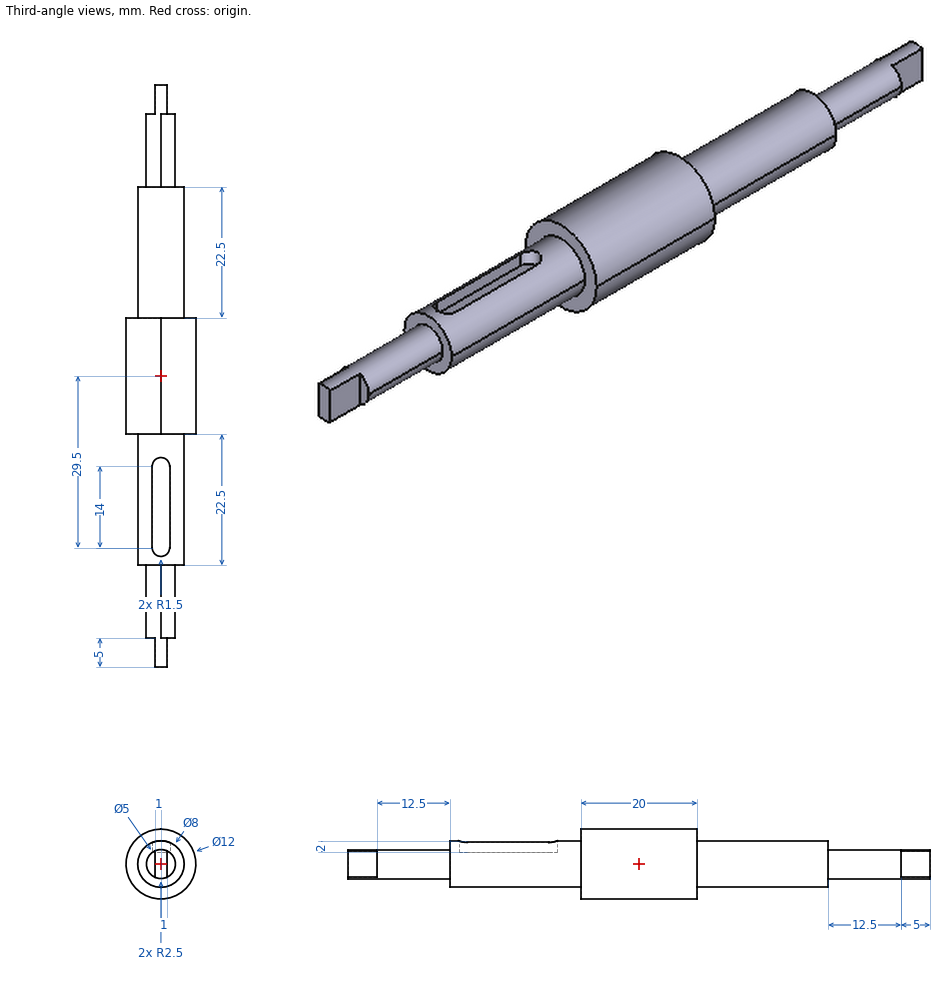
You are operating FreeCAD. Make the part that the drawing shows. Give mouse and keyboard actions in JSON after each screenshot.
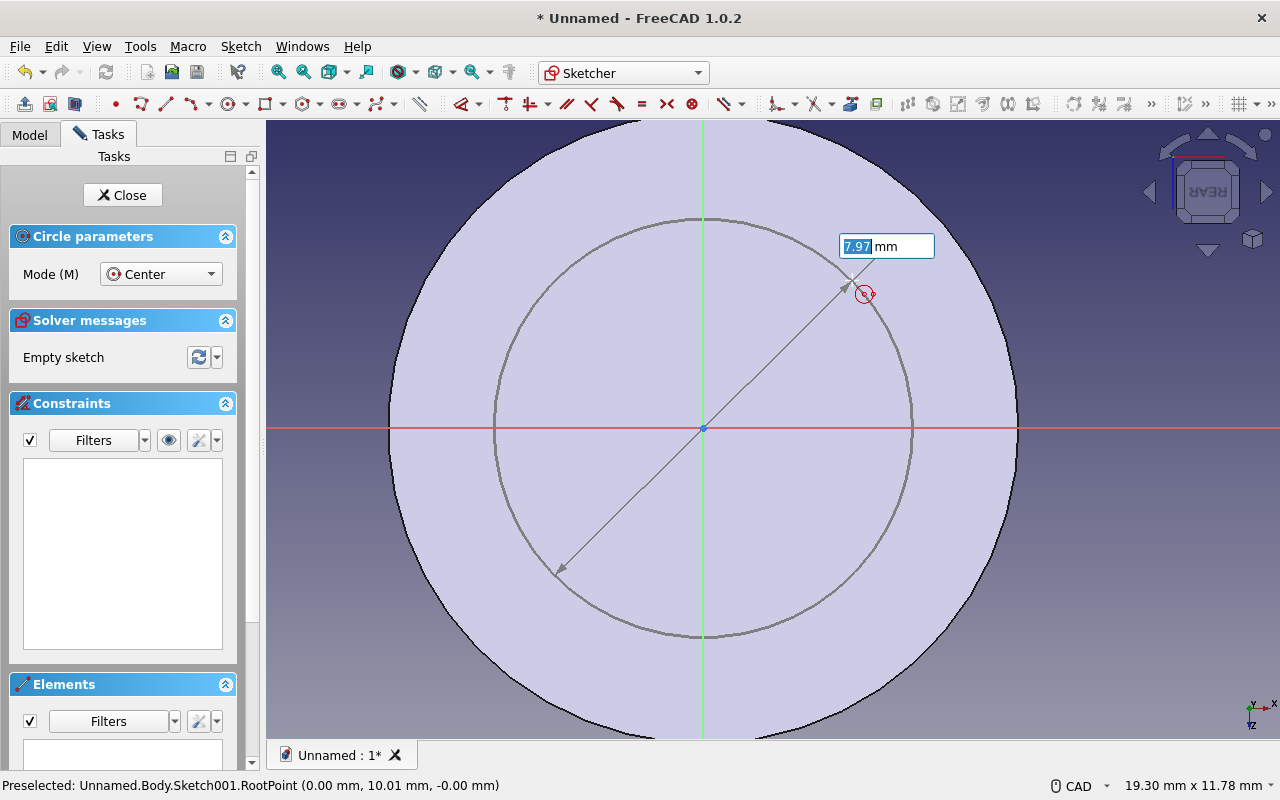
{"action": "type", "text": "8"}
{"action": "key", "text": "Return"}
{"action": "key", "text": "Escape"}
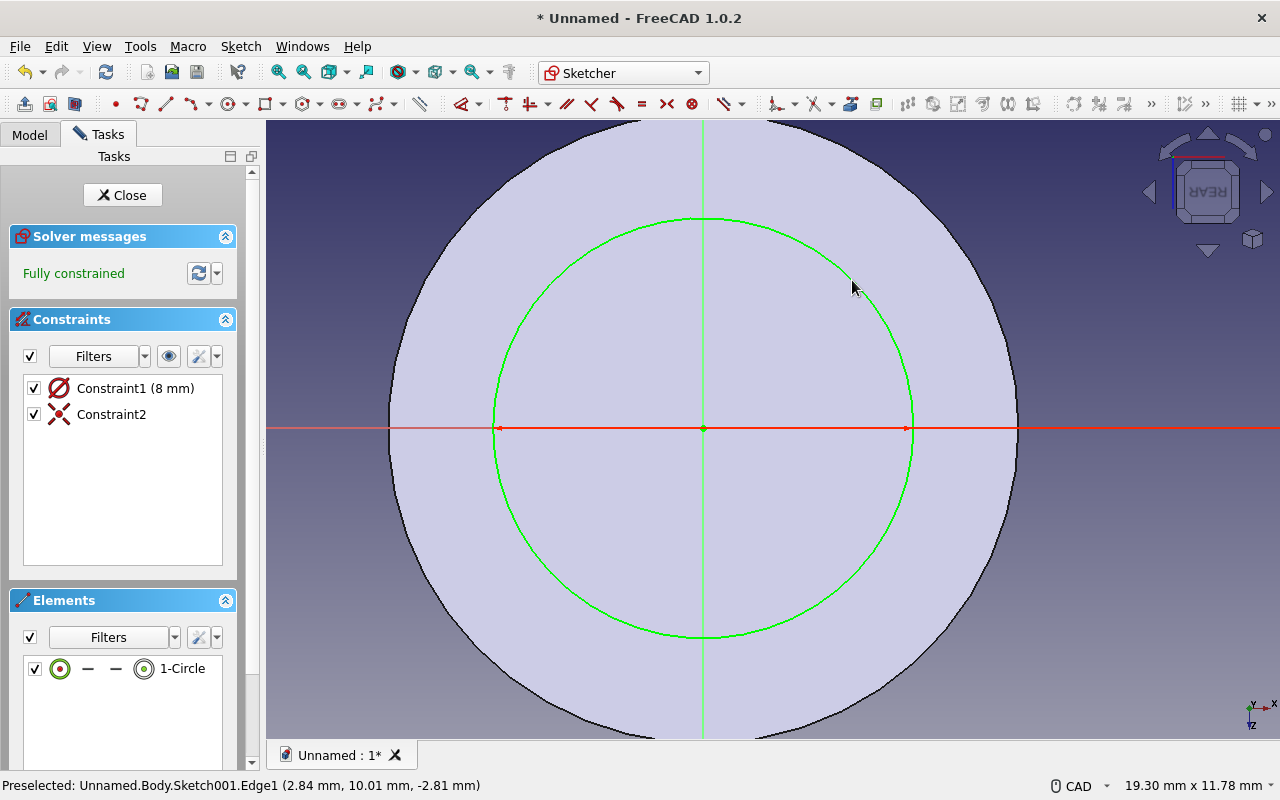
{"action": "left_click", "coordinate": [123, 195]}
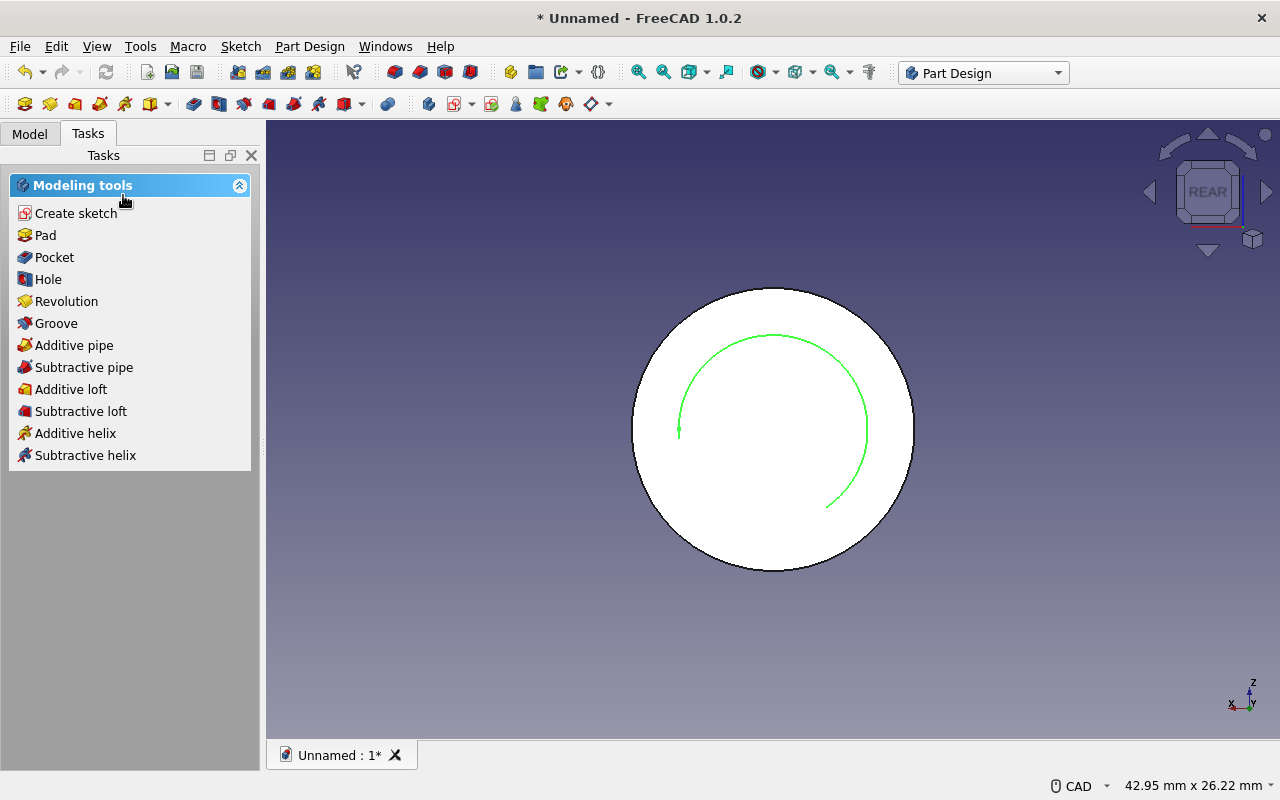
{"action": "left_click", "coordinate": [25, 104]}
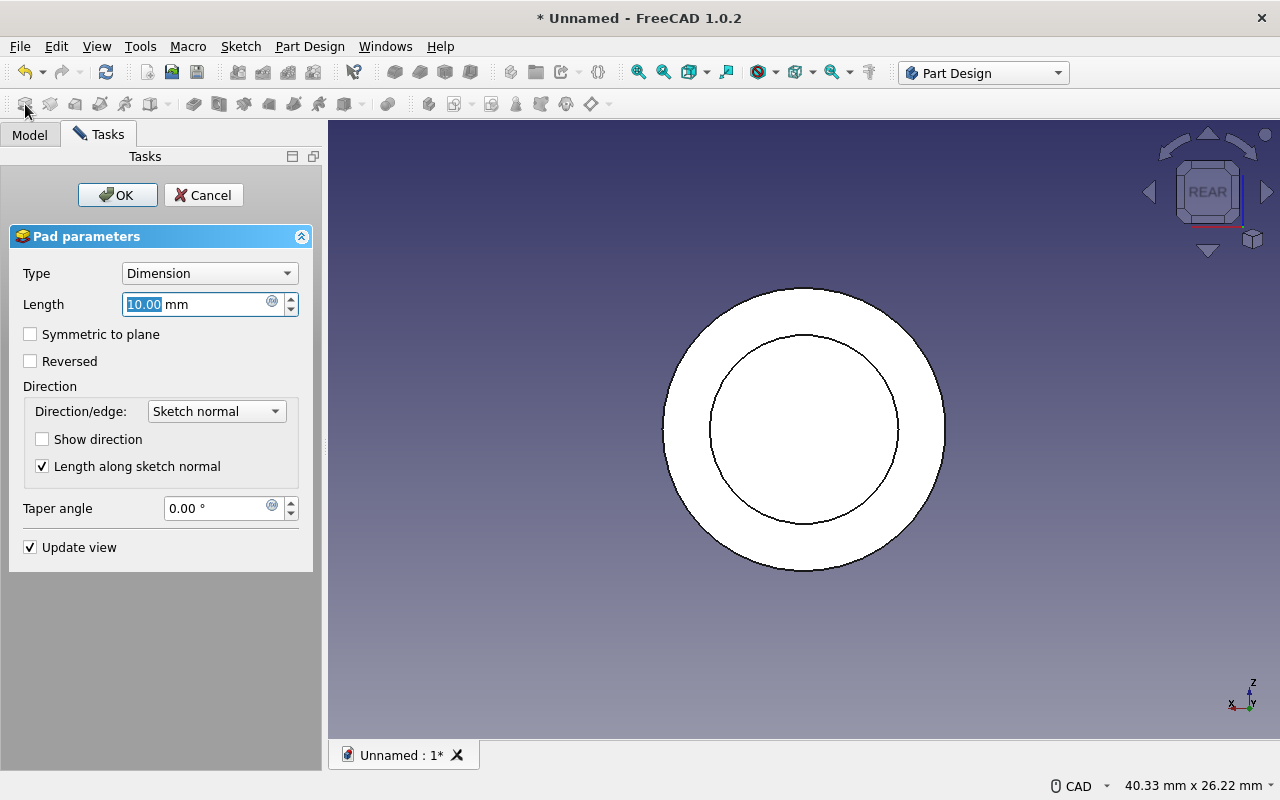
{"action": "type", "text": "22.5"}
{"action": "key", "text": "Tab"}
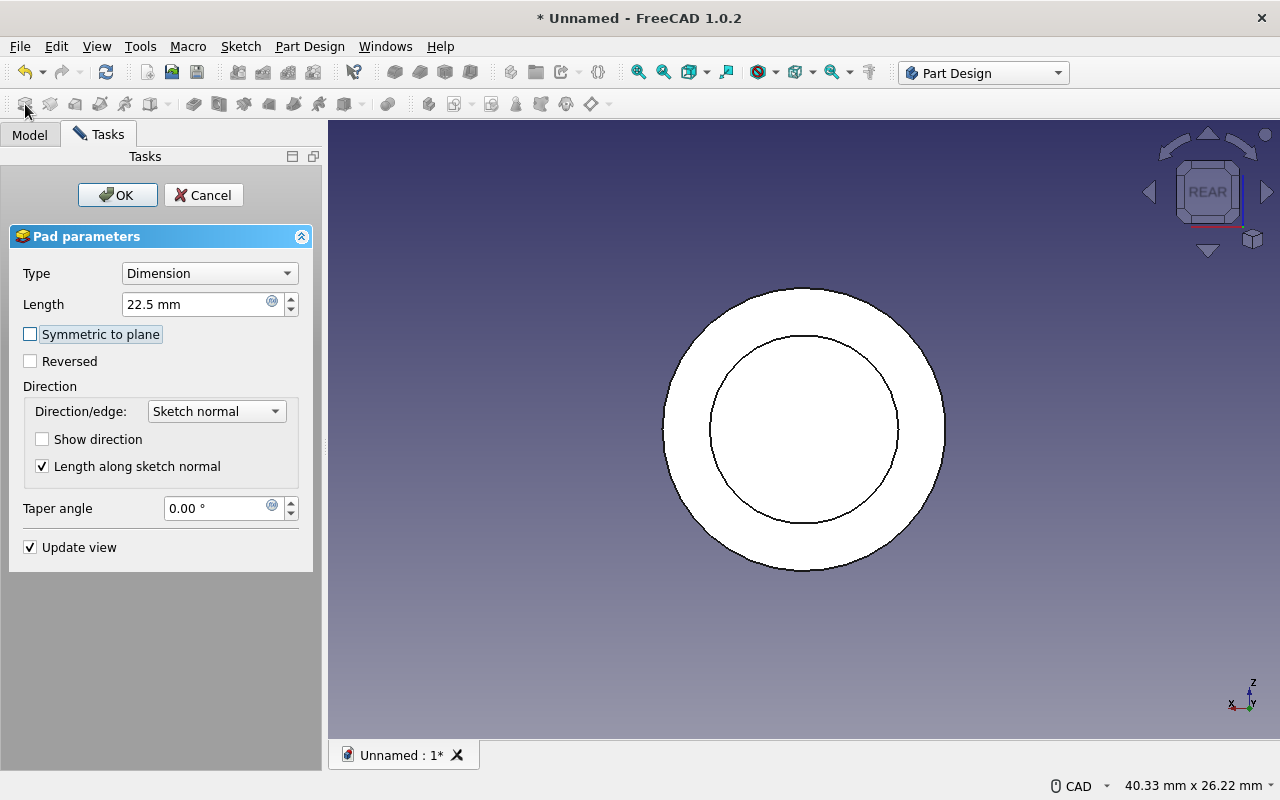
{"action": "left_click", "coordinate": [118, 195]}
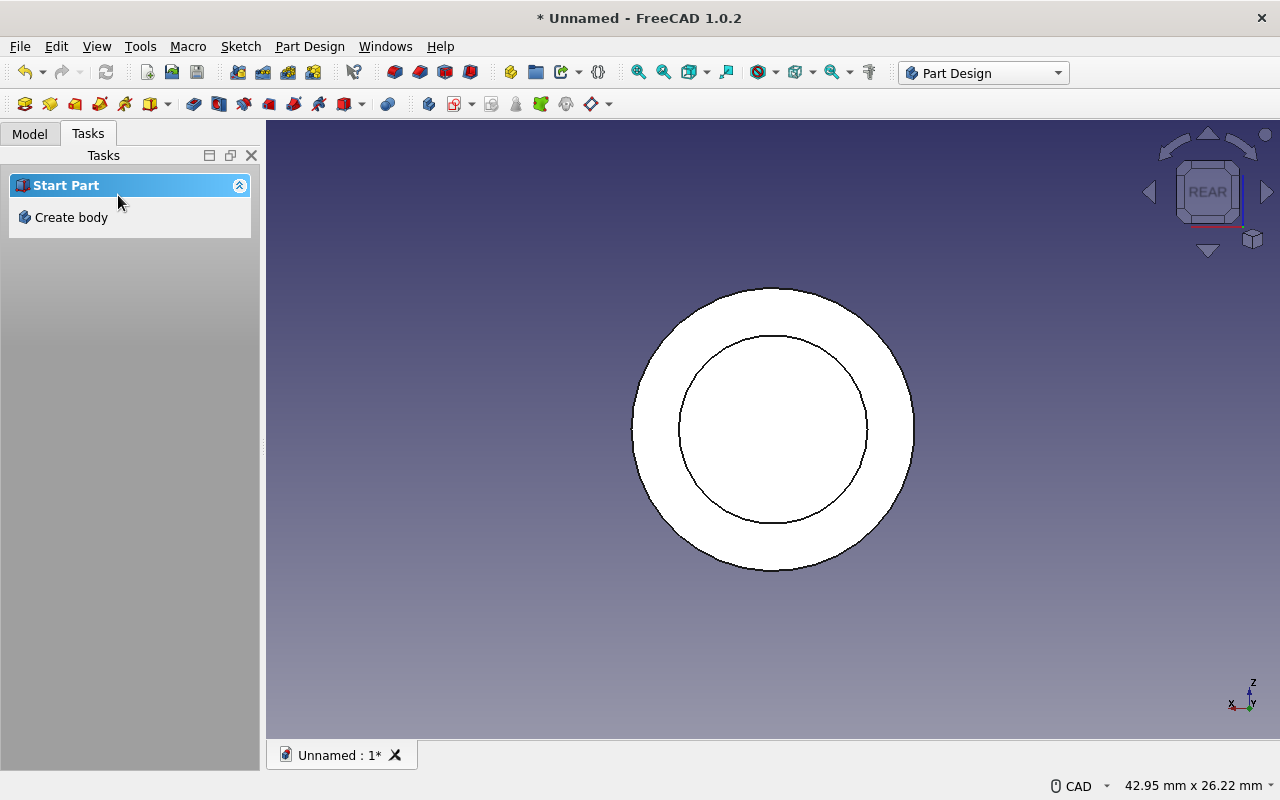
{"action": "left_click", "coordinate": [773, 428]}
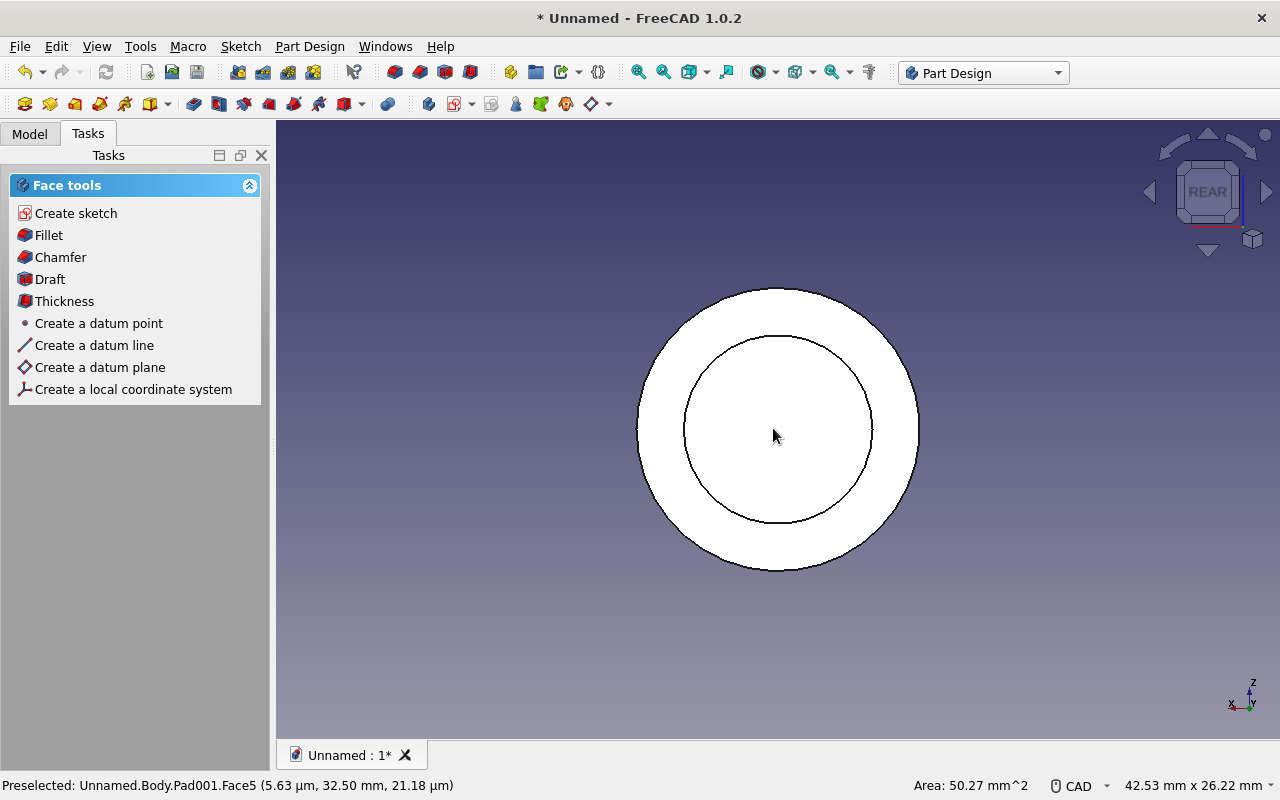
{"action": "left_click", "coordinate": [454, 104]}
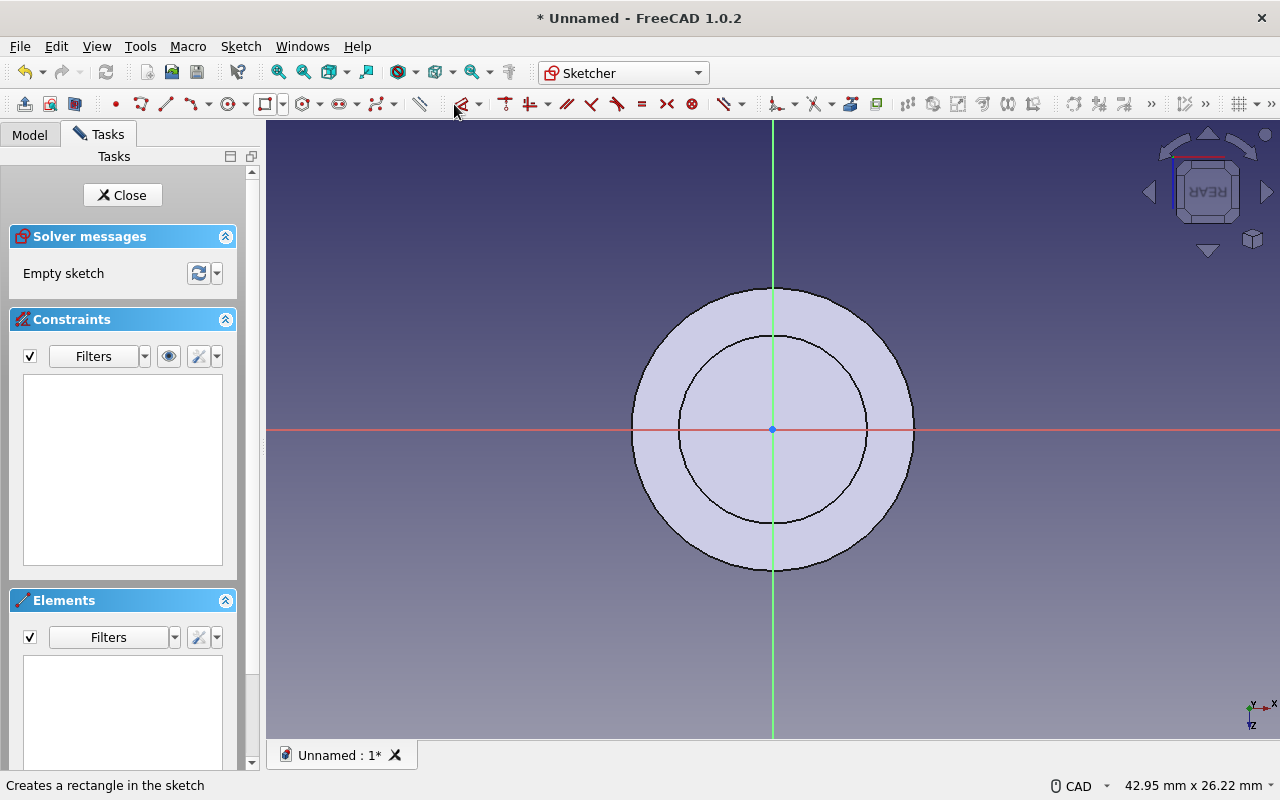
{"action": "scroll", "coordinate": [802, 429], "scroll_direction": "up", "scroll_amount": 6}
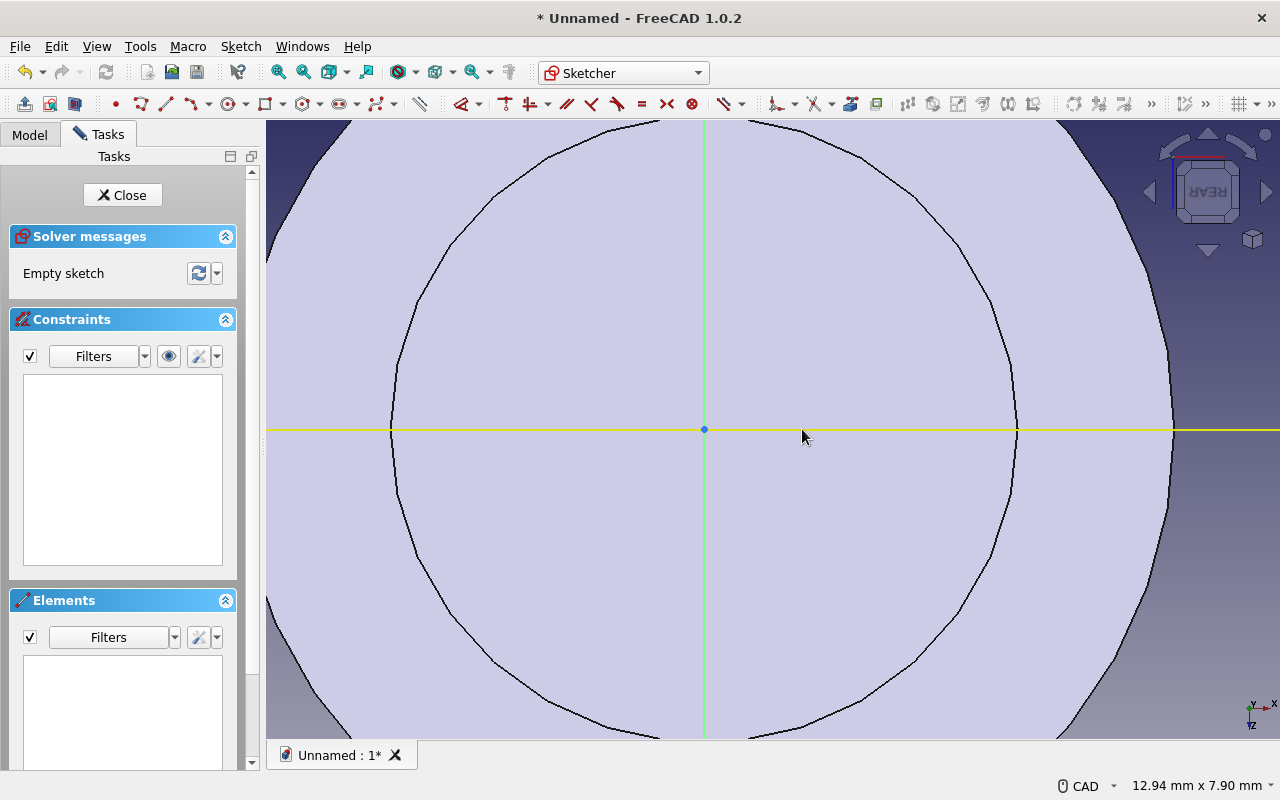
{"action": "key", "text": "g c"}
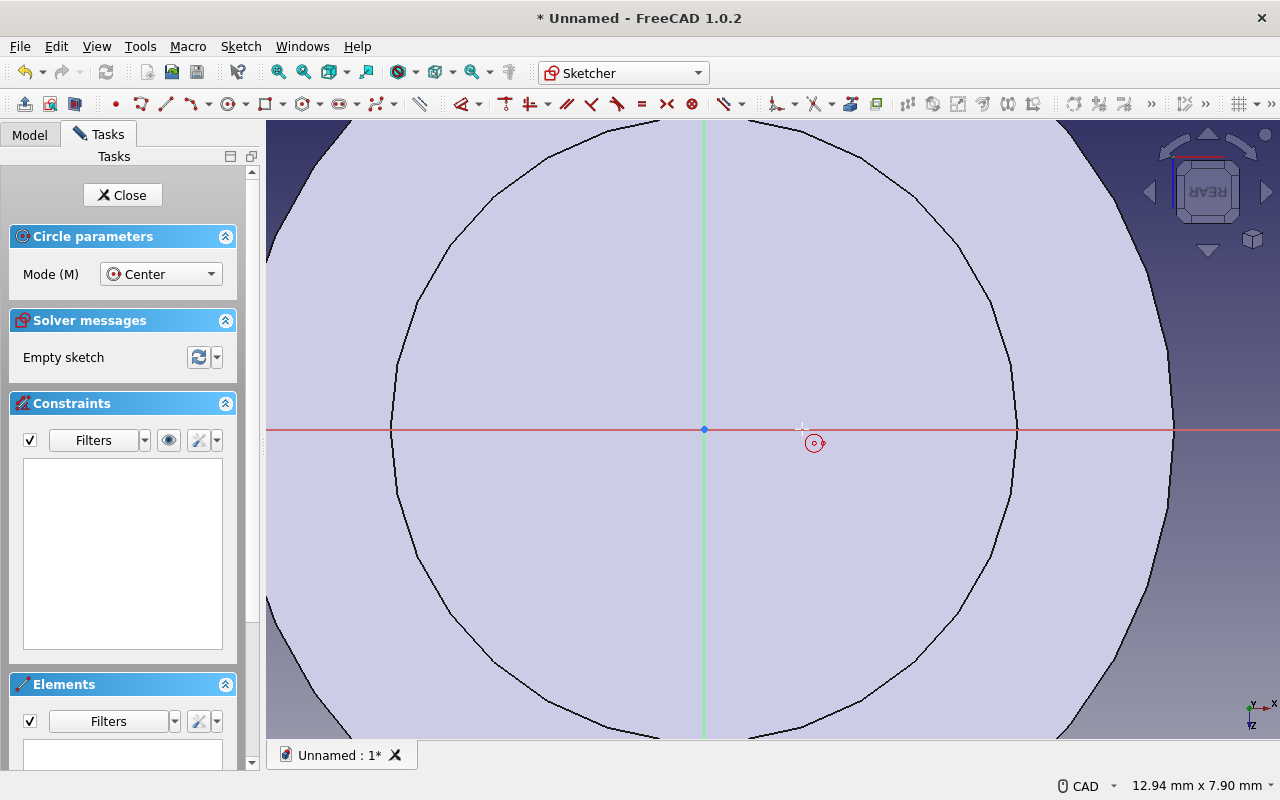
{"action": "left_click", "coordinate": [704, 429]}
{"action": "mouse_move", "coordinate": [843, 291]}